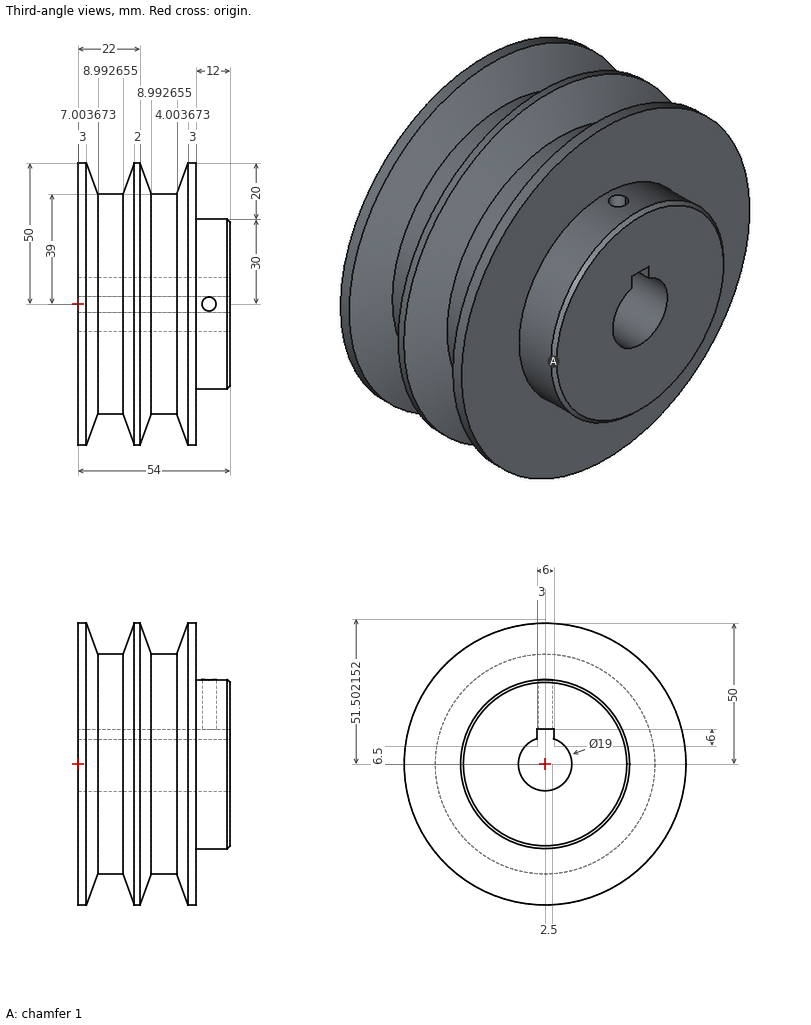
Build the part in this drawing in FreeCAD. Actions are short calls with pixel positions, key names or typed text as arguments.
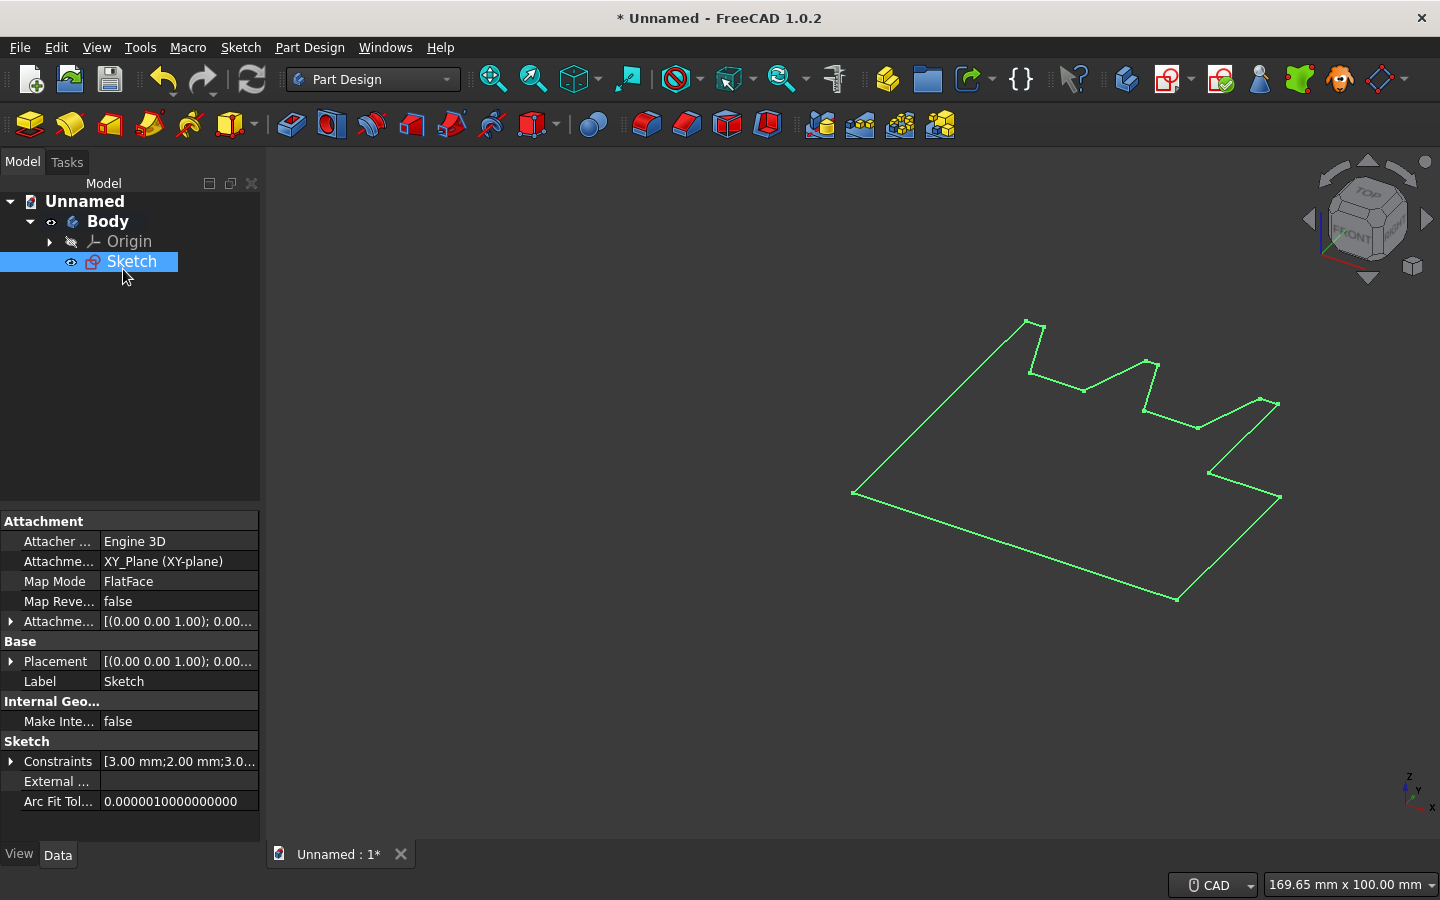
click(70, 124)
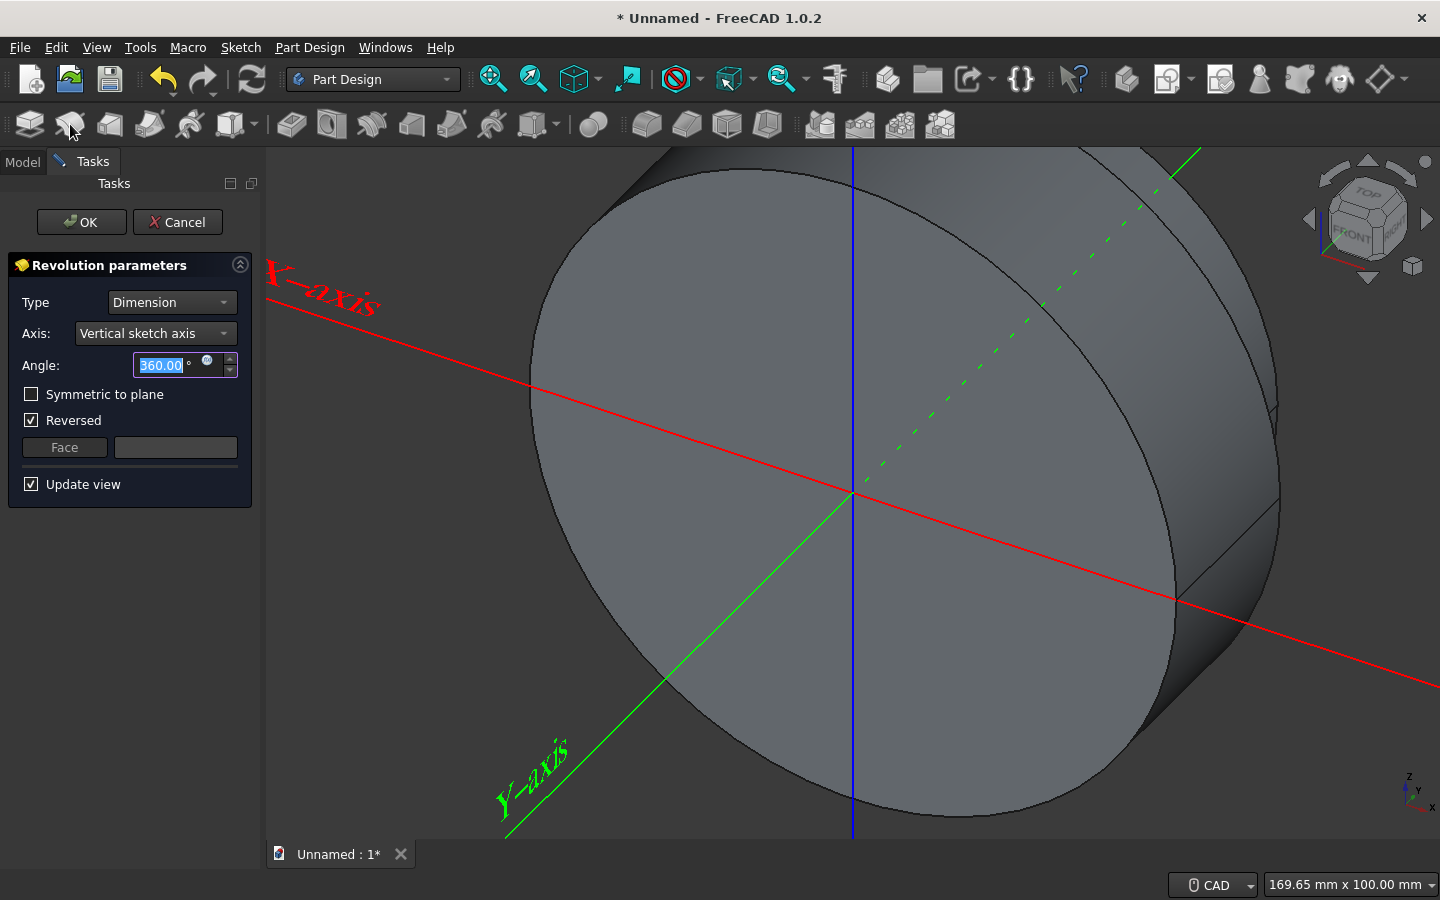
click(156, 334)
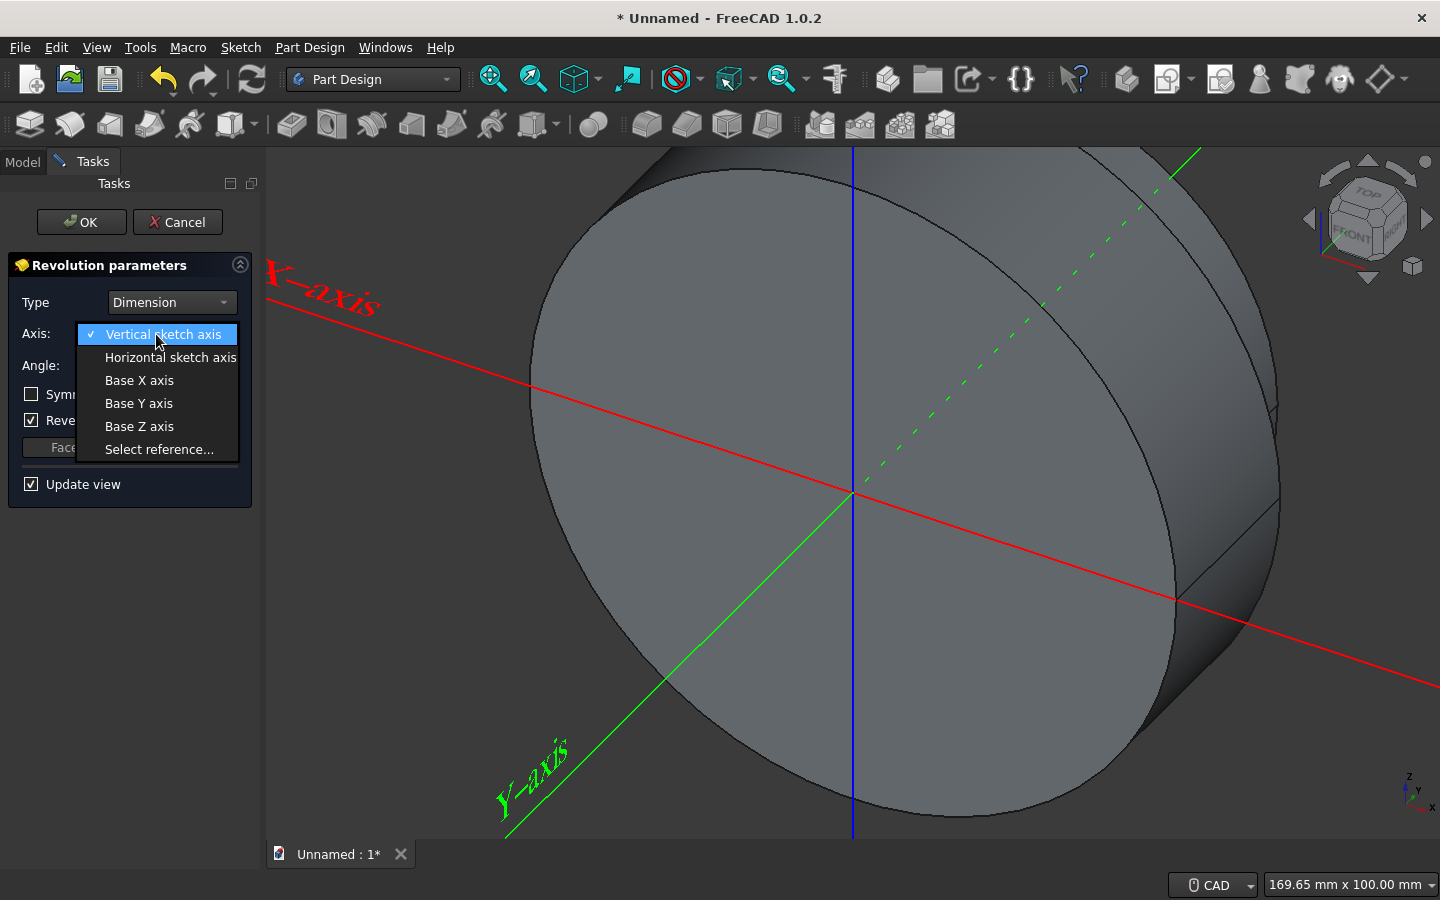
click(156, 358)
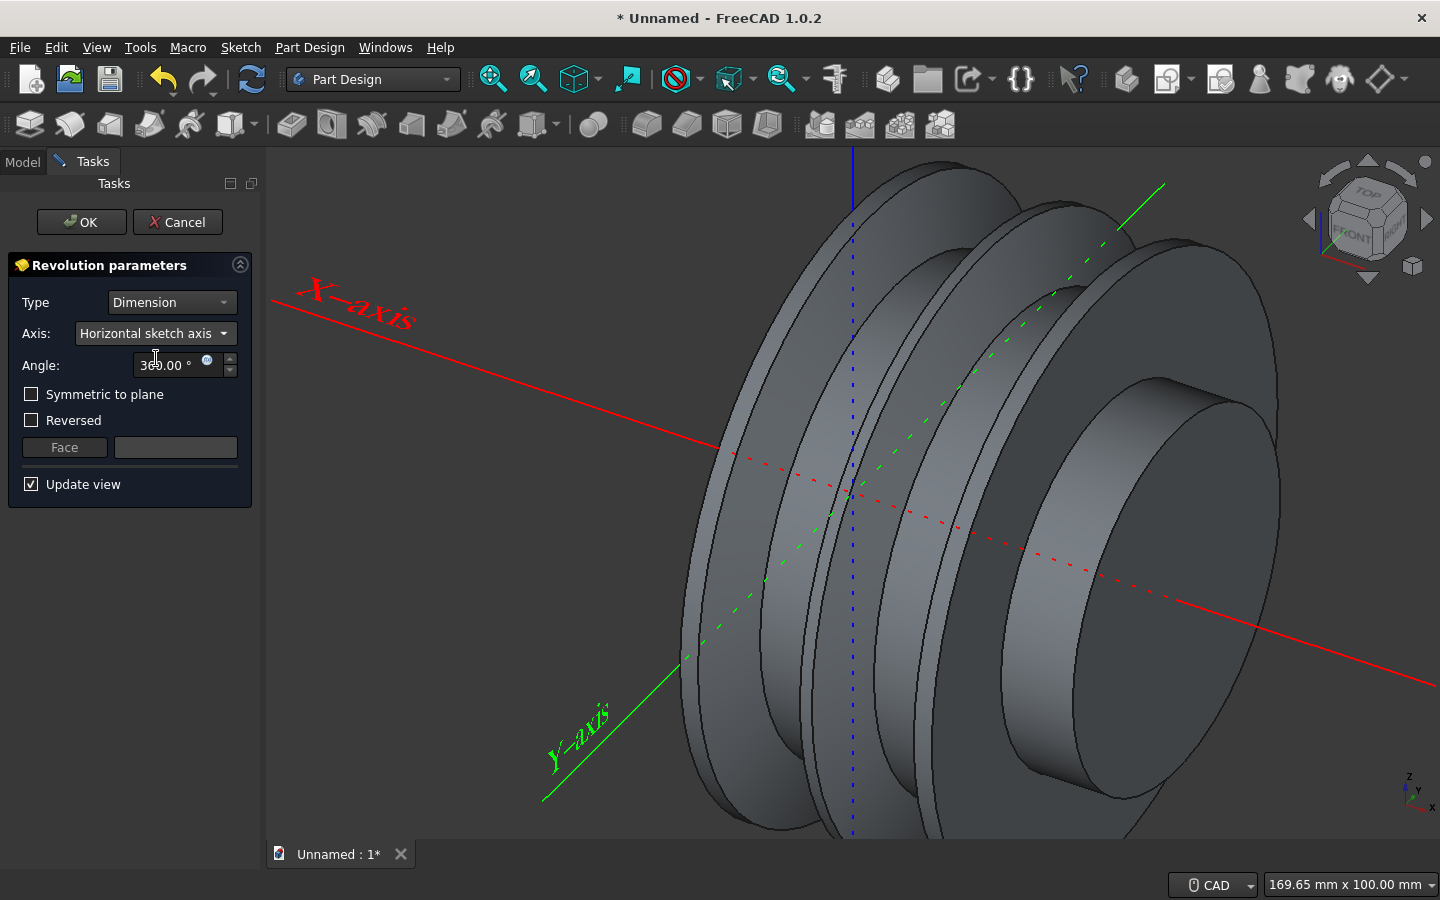
click(82, 222)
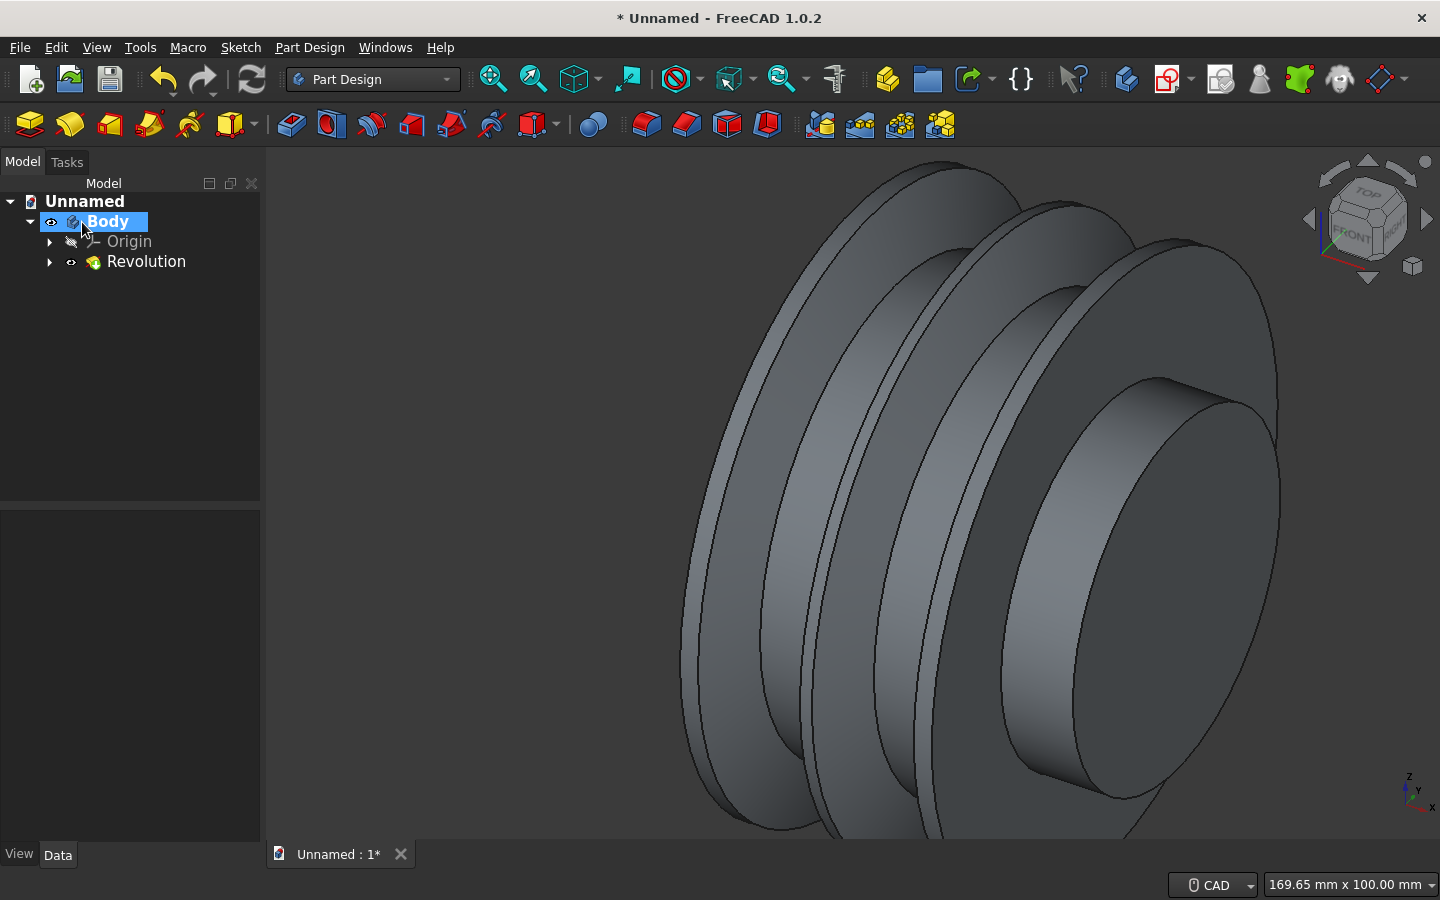
click(494, 80)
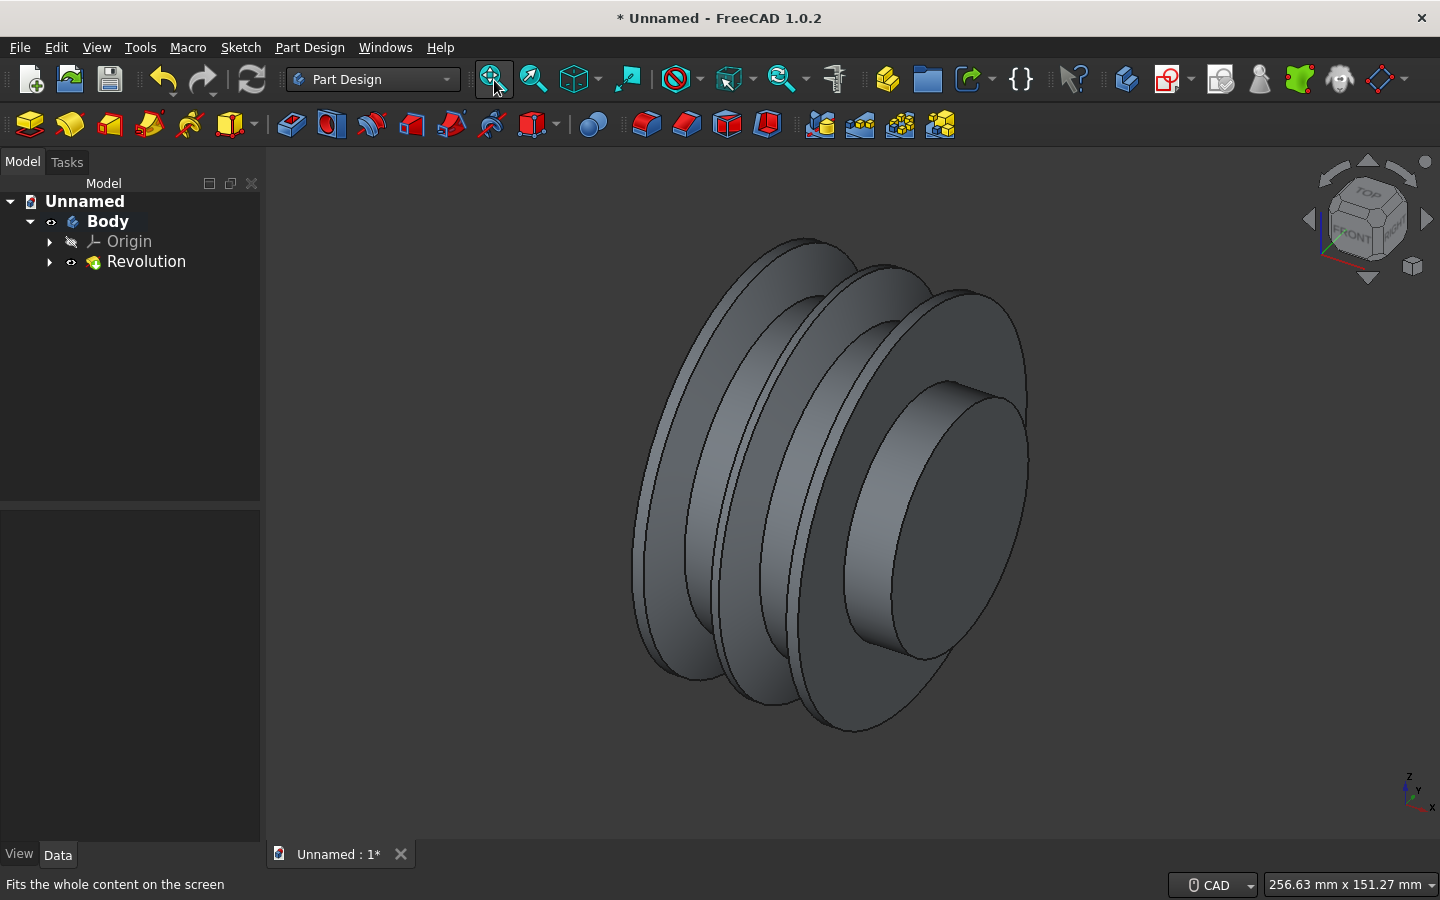
click(960, 527)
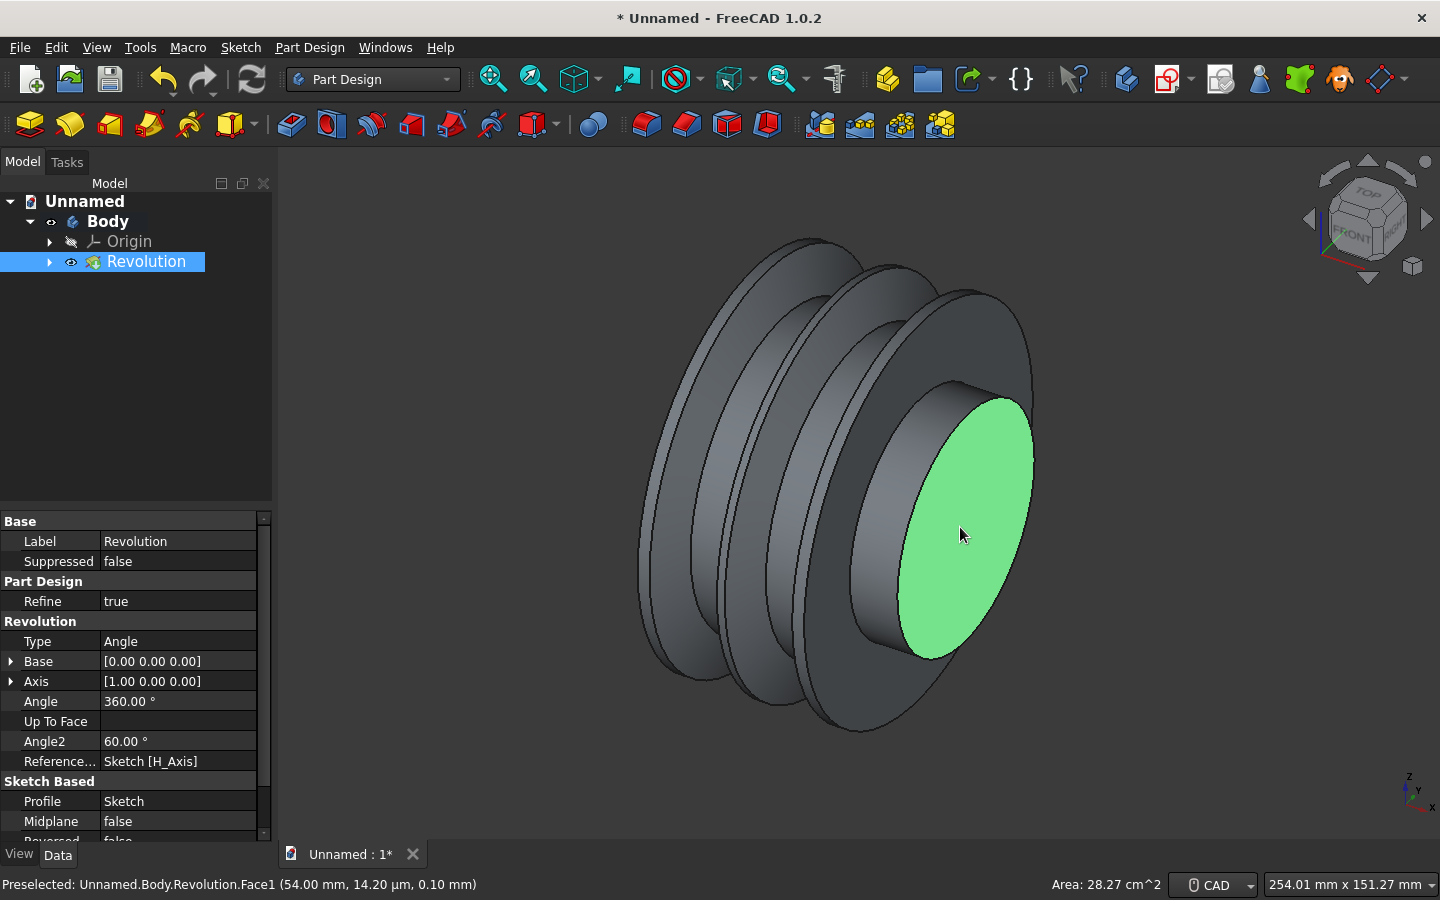
click(1168, 80)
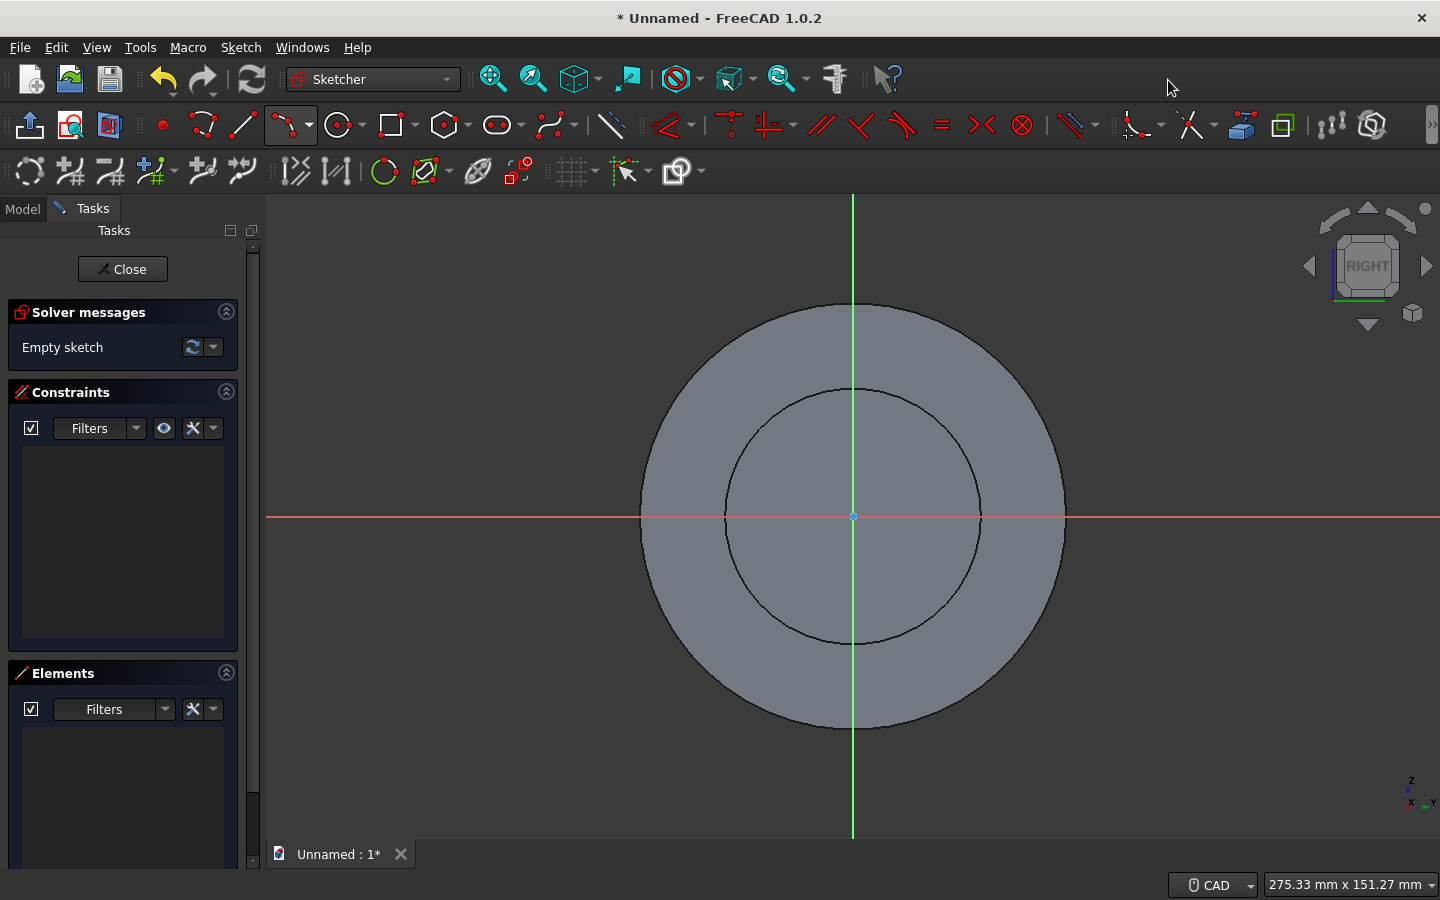
scroll(870, 516, up, 8)